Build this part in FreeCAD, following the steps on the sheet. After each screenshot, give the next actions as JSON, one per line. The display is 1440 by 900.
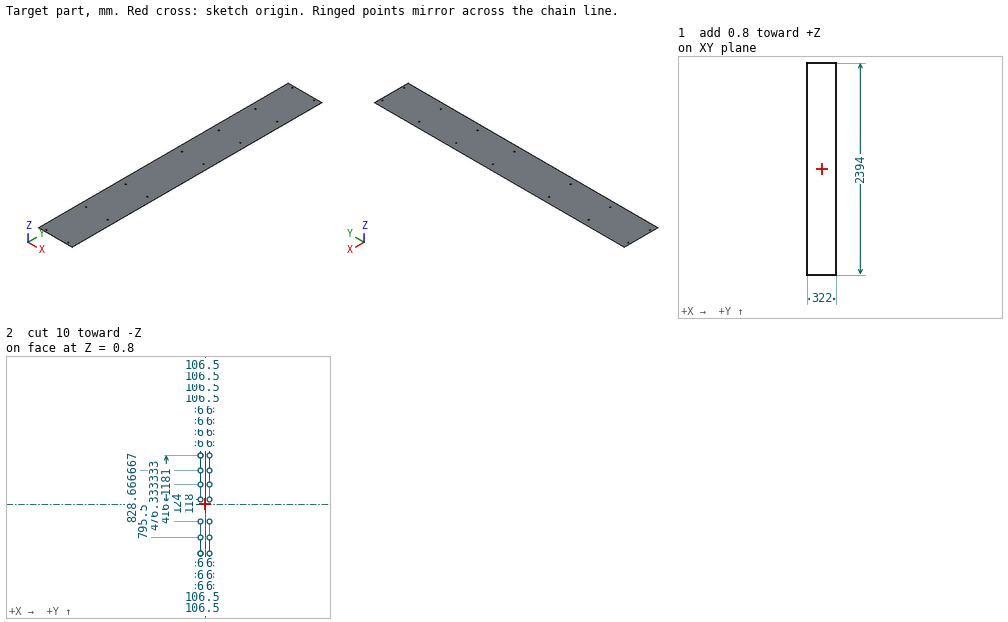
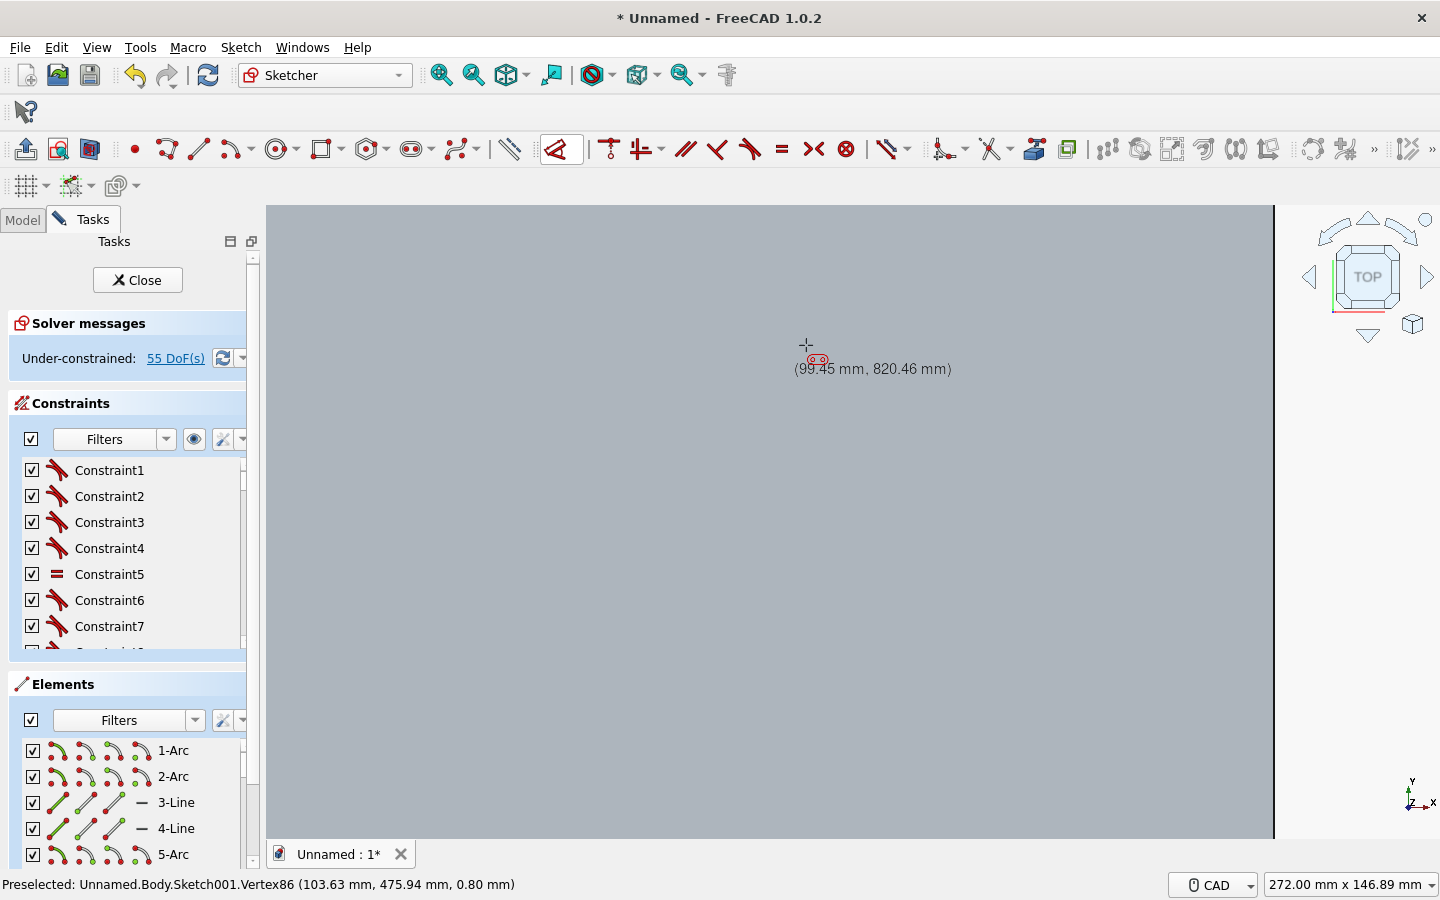
{"action": "scroll", "coordinate": [806, 345], "scroll_direction": "down", "scroll_amount": 18}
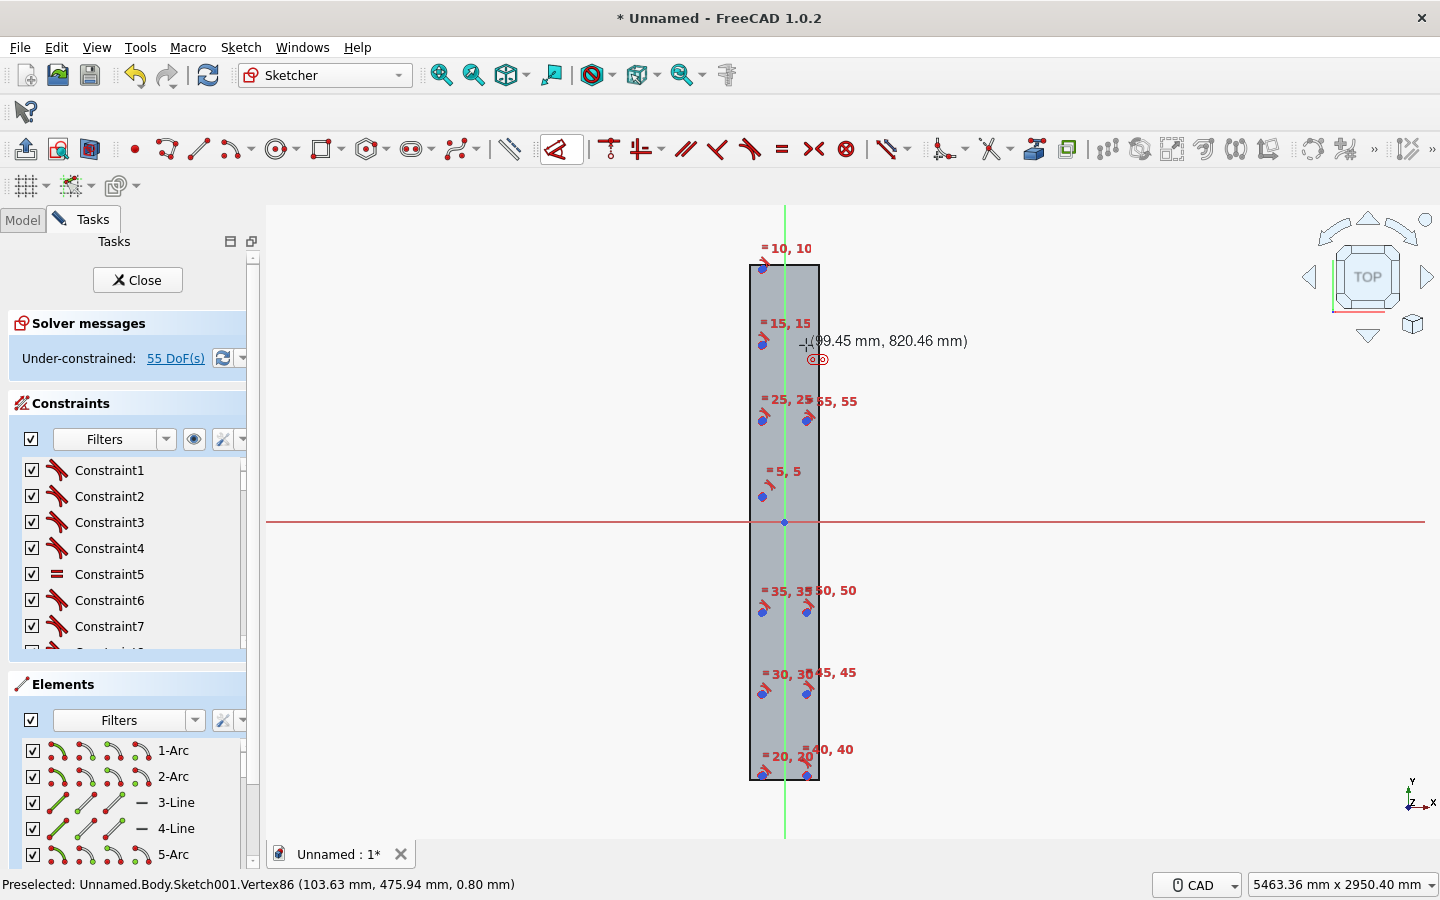
{"action": "left_click", "coordinate": [806, 345]}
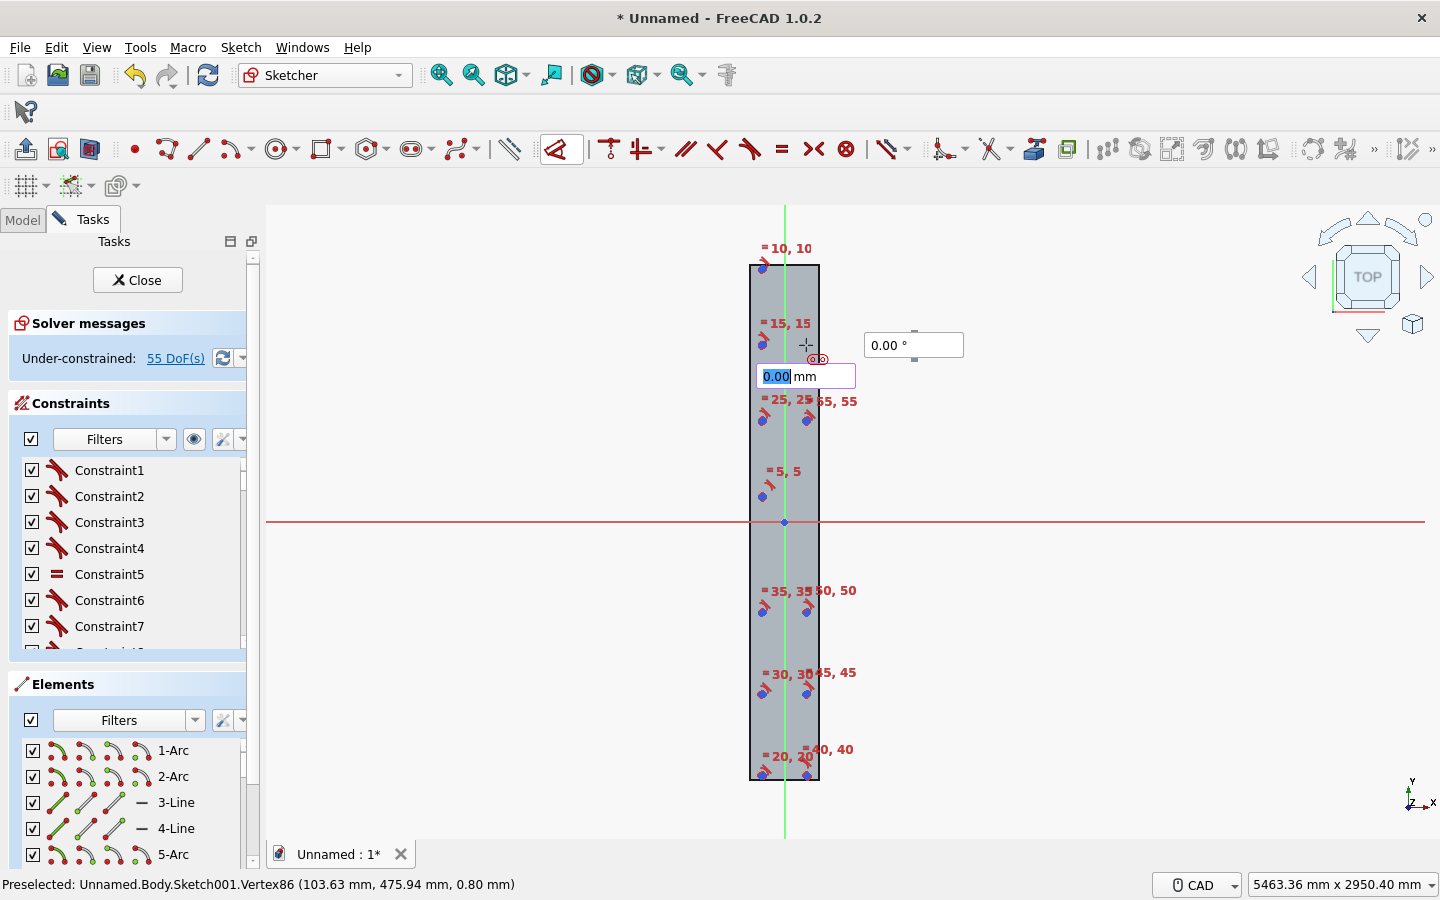
{"action": "scroll", "coordinate": [808, 345], "scroll_direction": "up", "scroll_amount": 13}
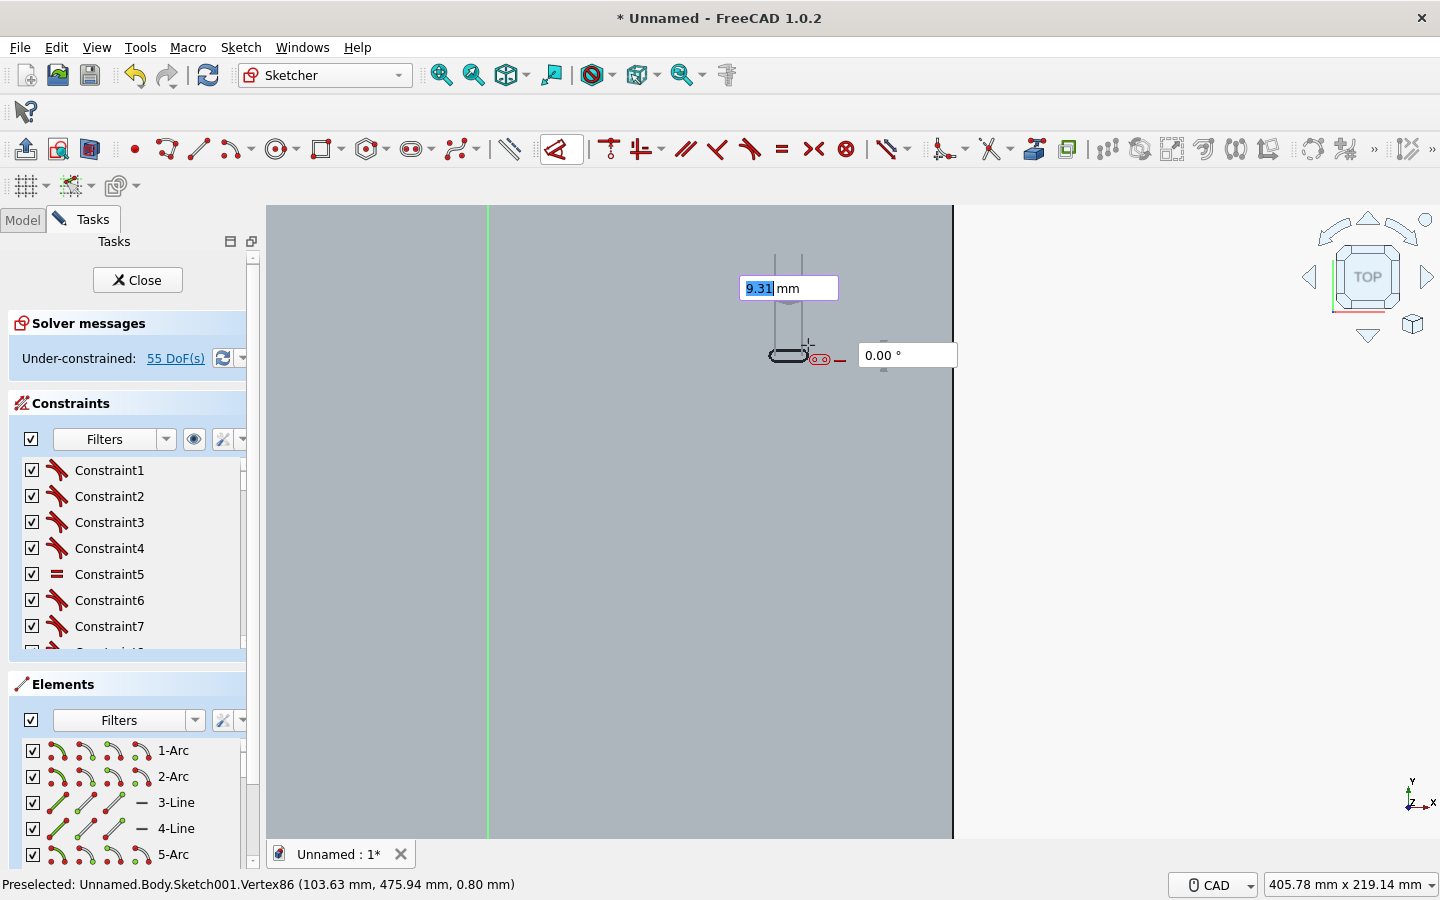
{"action": "left_click", "coordinate": [796, 342]}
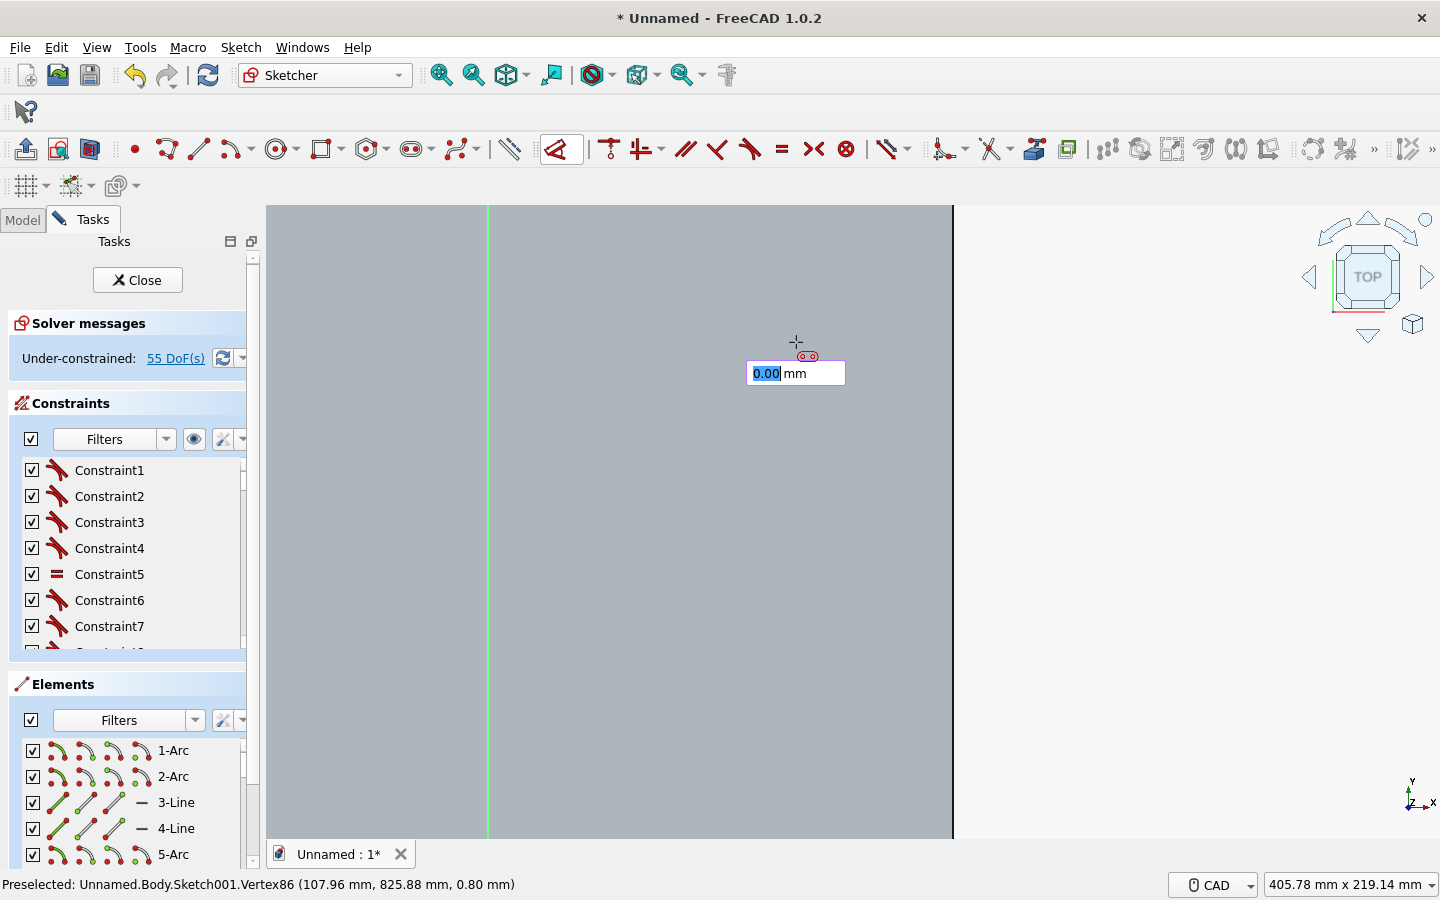
{"action": "scroll", "coordinate": [787, 332], "scroll_direction": "up", "scroll_amount": 4}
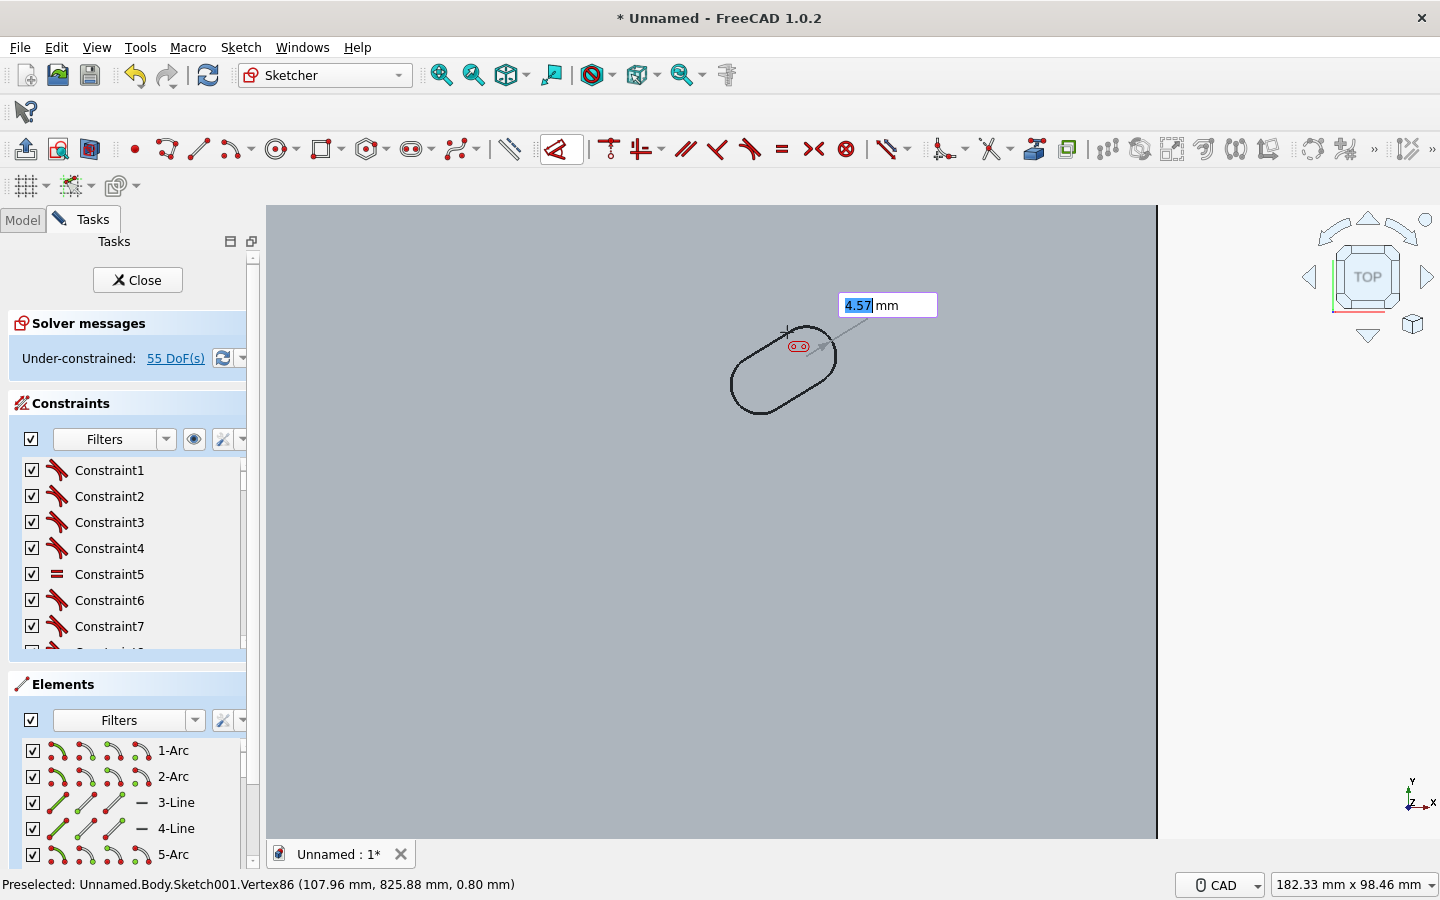
{"action": "left_click", "coordinate": [787, 332]}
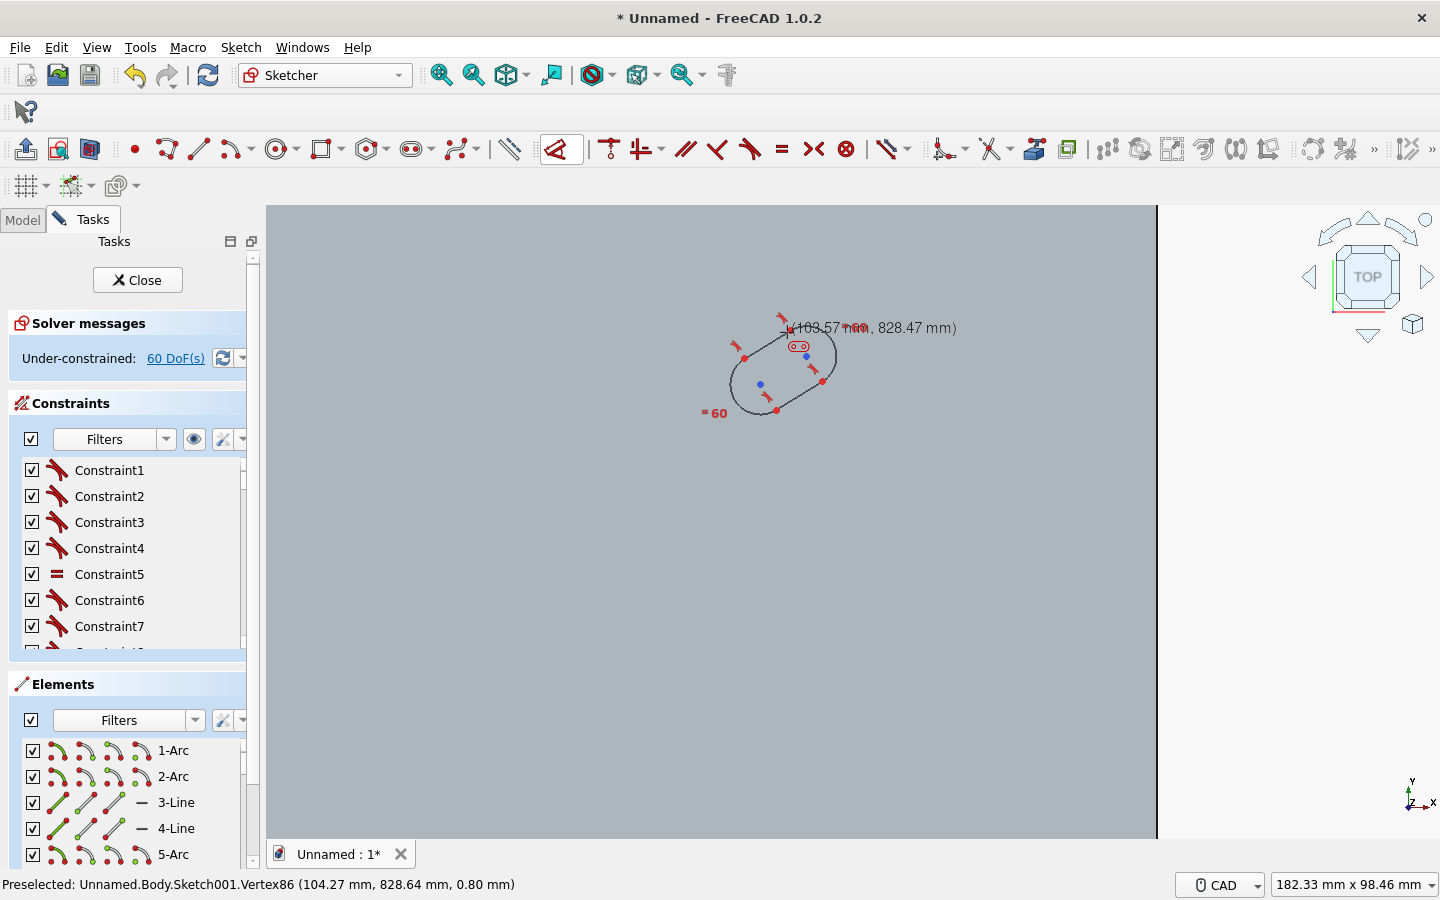
{"action": "scroll", "coordinate": [807, 344], "scroll_direction": "down", "scroll_amount": 17}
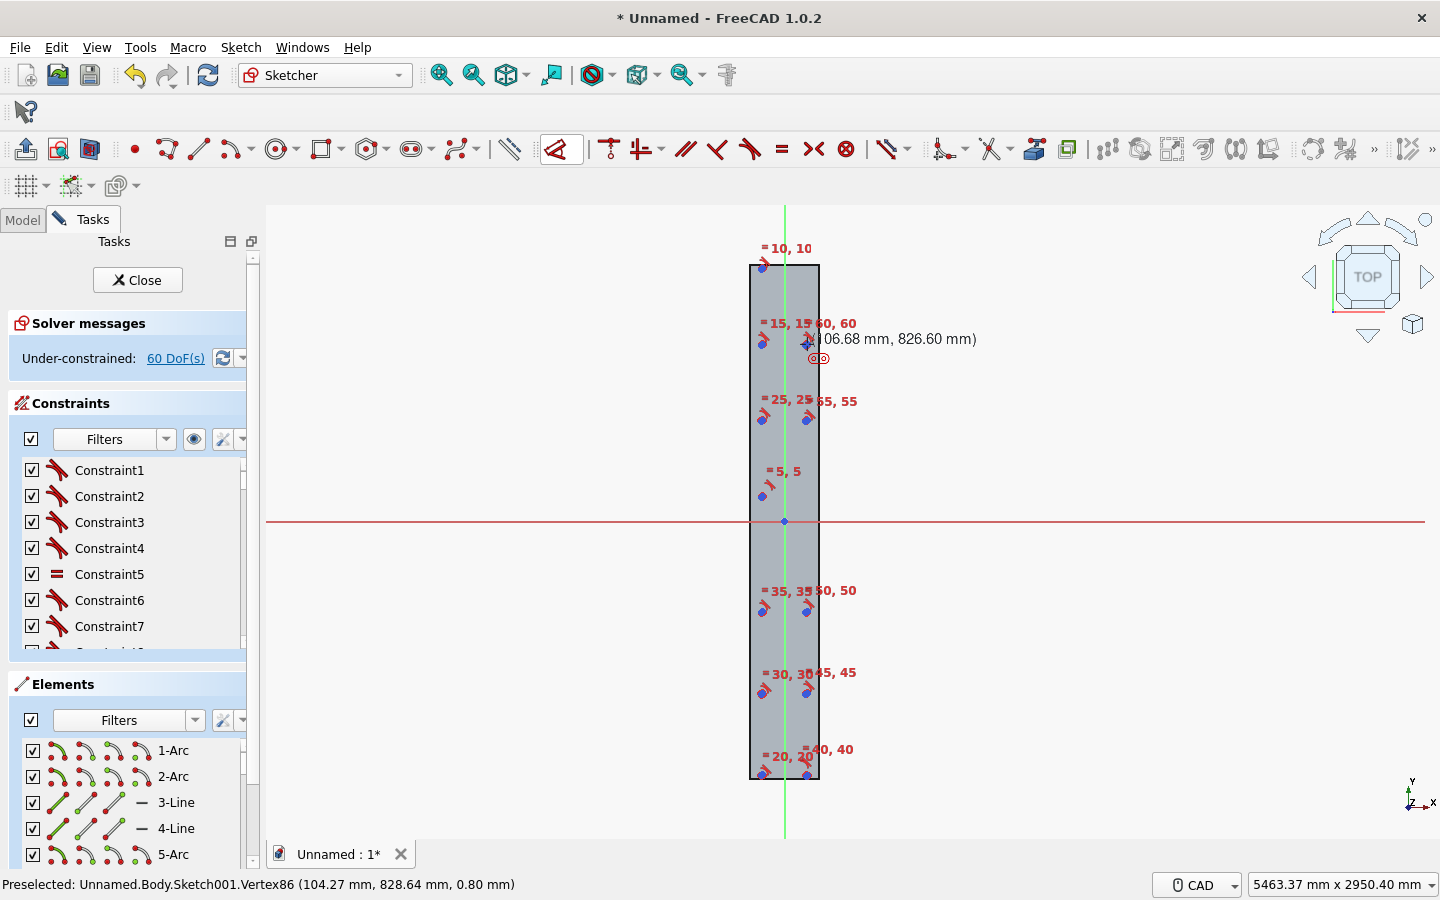
{"action": "scroll", "coordinate": [806, 269], "scroll_direction": "up", "scroll_amount": 18}